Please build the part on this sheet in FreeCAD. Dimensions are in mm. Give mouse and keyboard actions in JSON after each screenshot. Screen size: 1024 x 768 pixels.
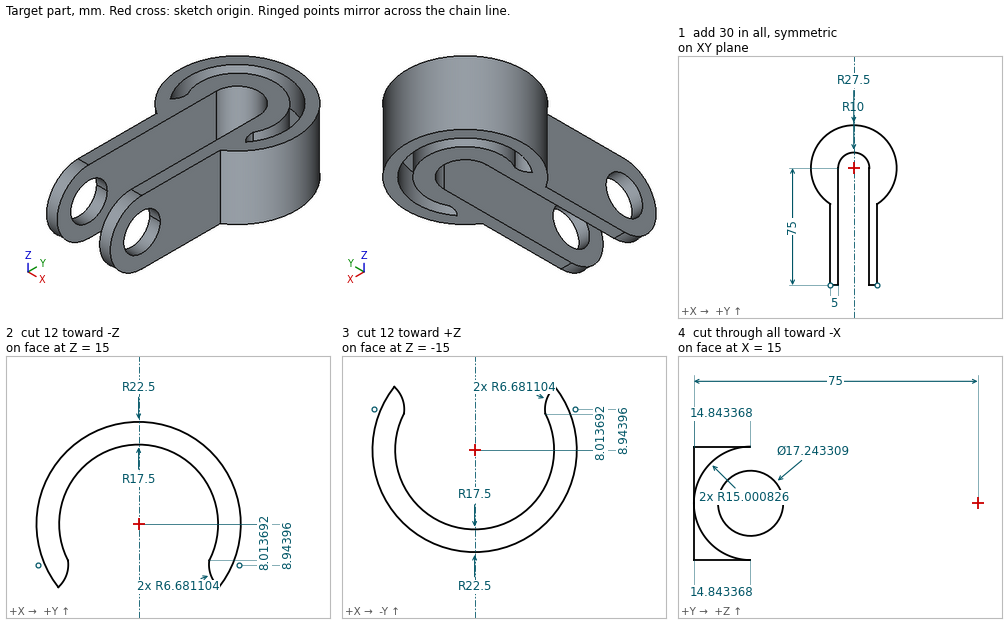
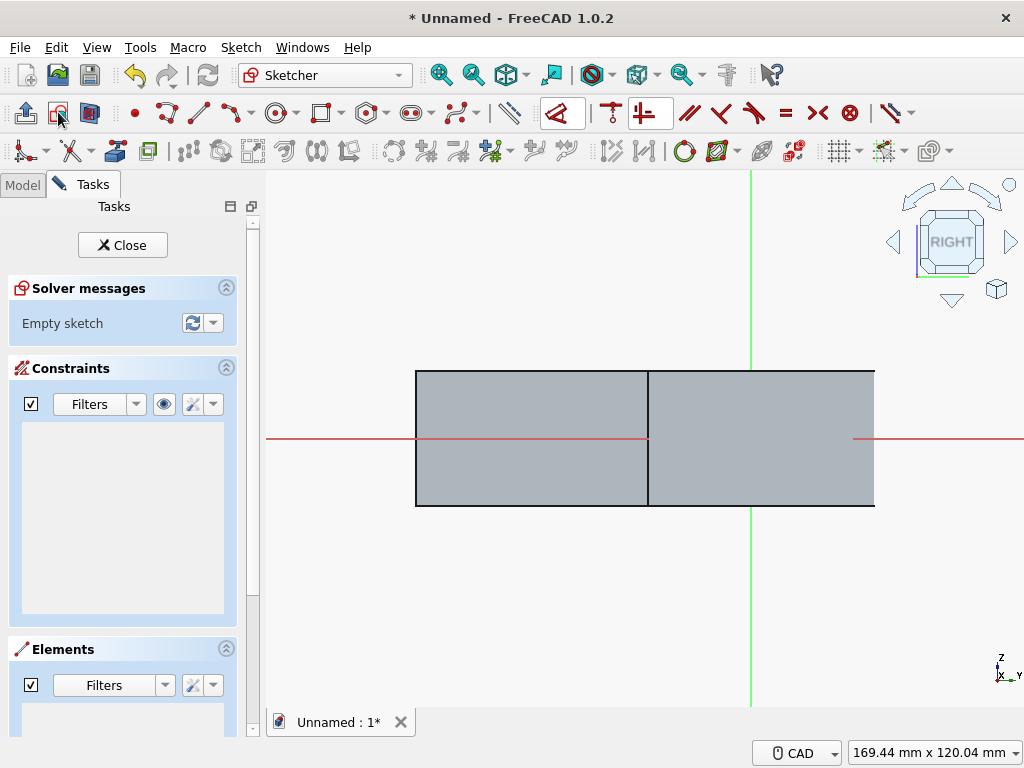
{"action": "left_click", "coordinate": [90, 114]}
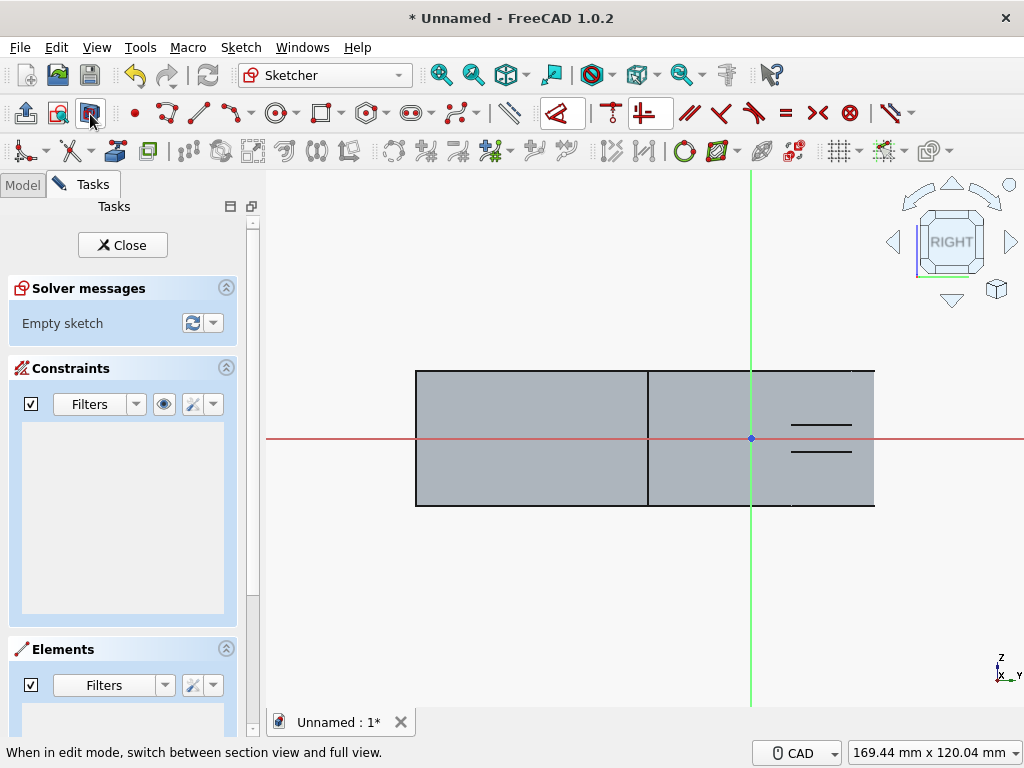
{"action": "scroll", "coordinate": [406, 439], "scroll_direction": "up", "scroll_amount": 5}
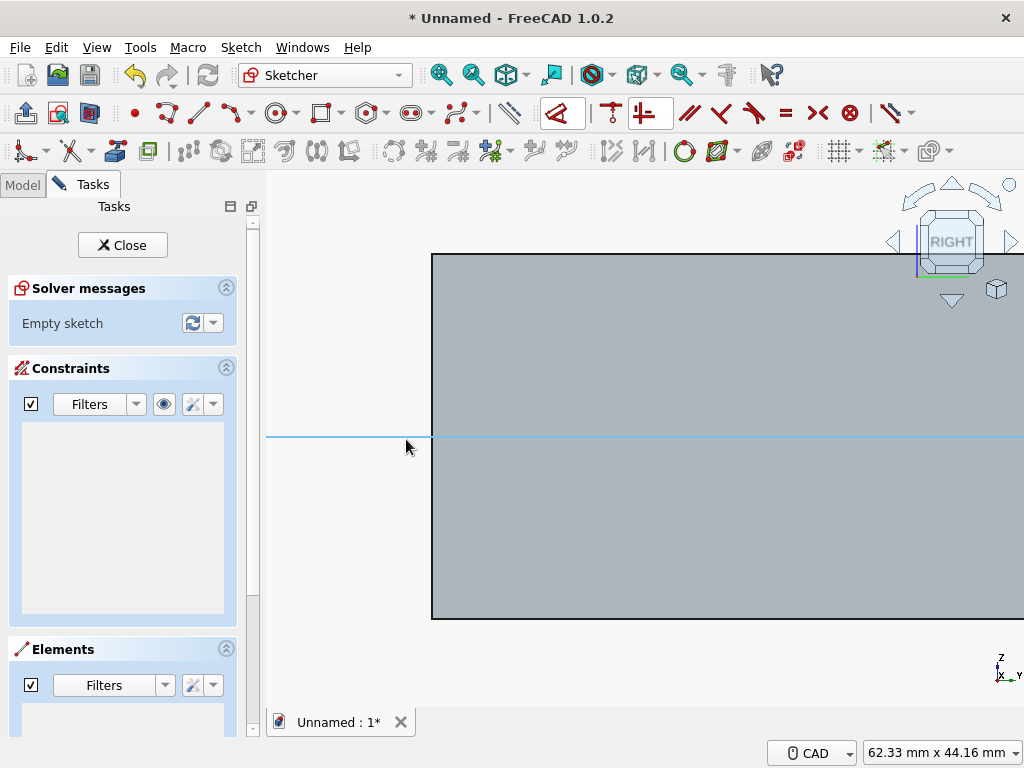
{"action": "left_click", "coordinate": [168, 114]}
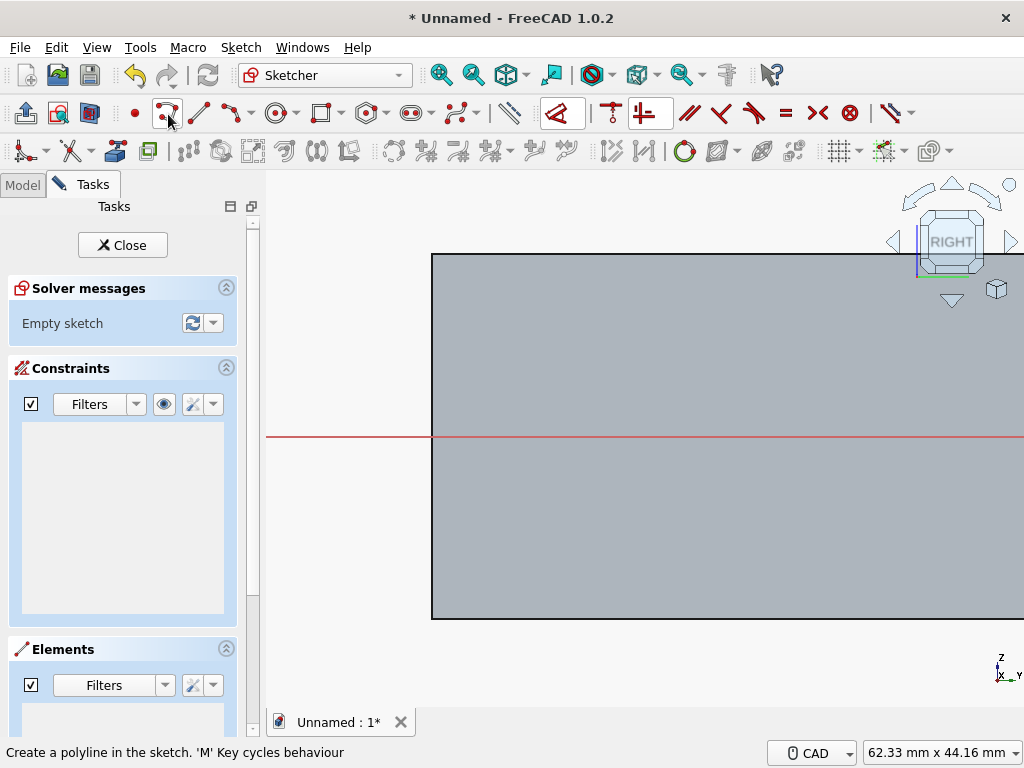
{"action": "left_click", "coordinate": [613, 254]}
{"action": "left_click", "coordinate": [432, 254]}
{"action": "left_click", "coordinate": [432, 437]}
{"action": "right_click", "coordinate": [432, 437]}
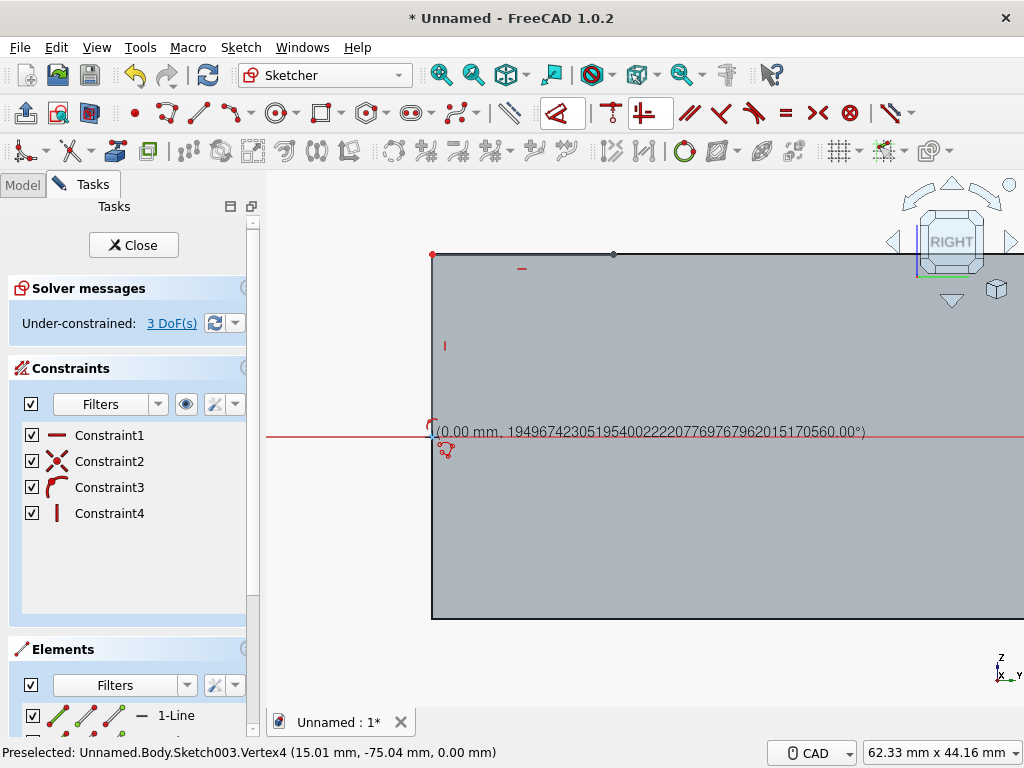
{"action": "left_click", "coordinate": [232, 114]}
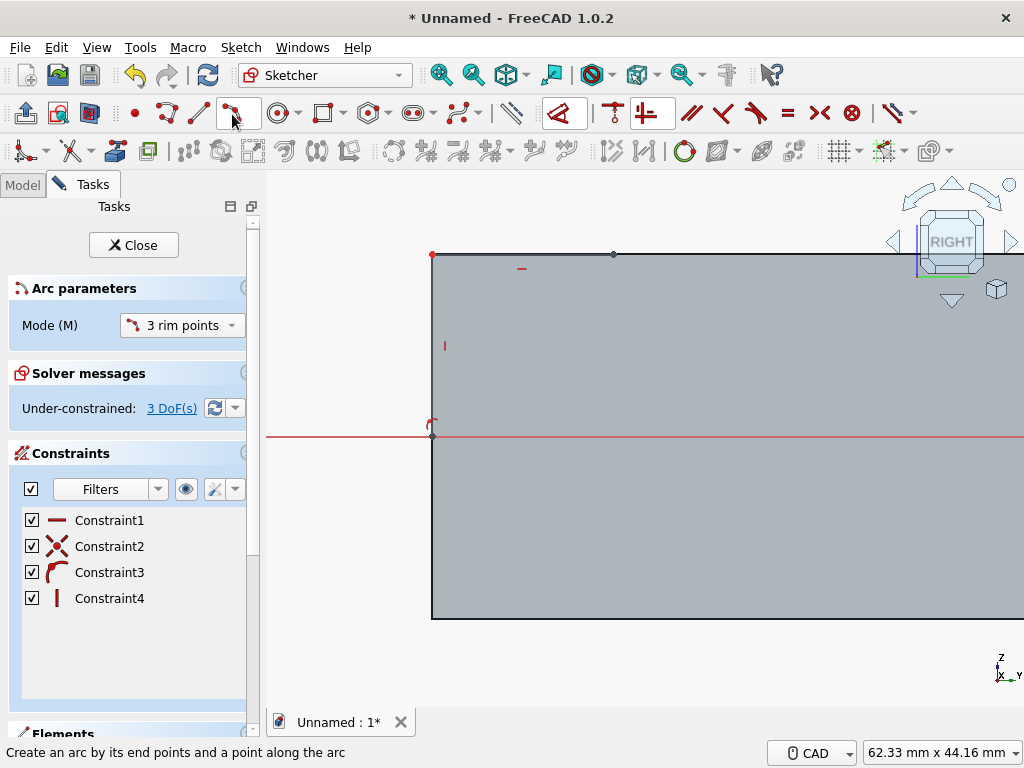
{"action": "left_click", "coordinate": [432, 437]}
{"action": "left_click", "coordinate": [613, 255]}
{"action": "left_click", "coordinate": [485, 308]}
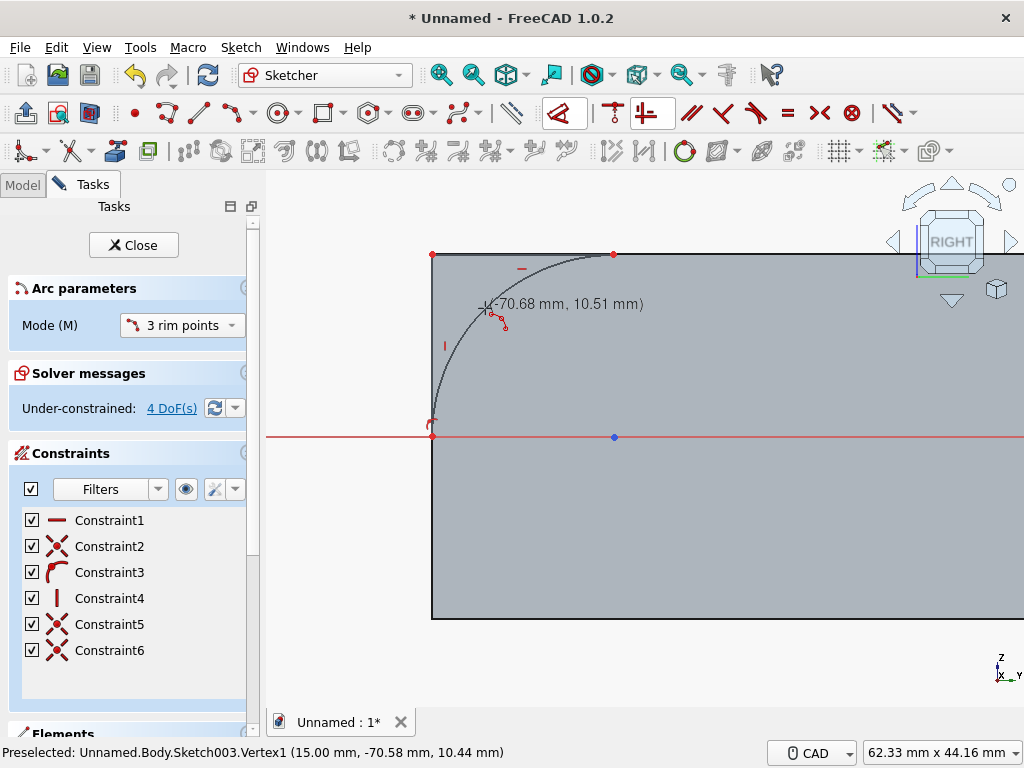
{"action": "left_click", "coordinate": [168, 114]}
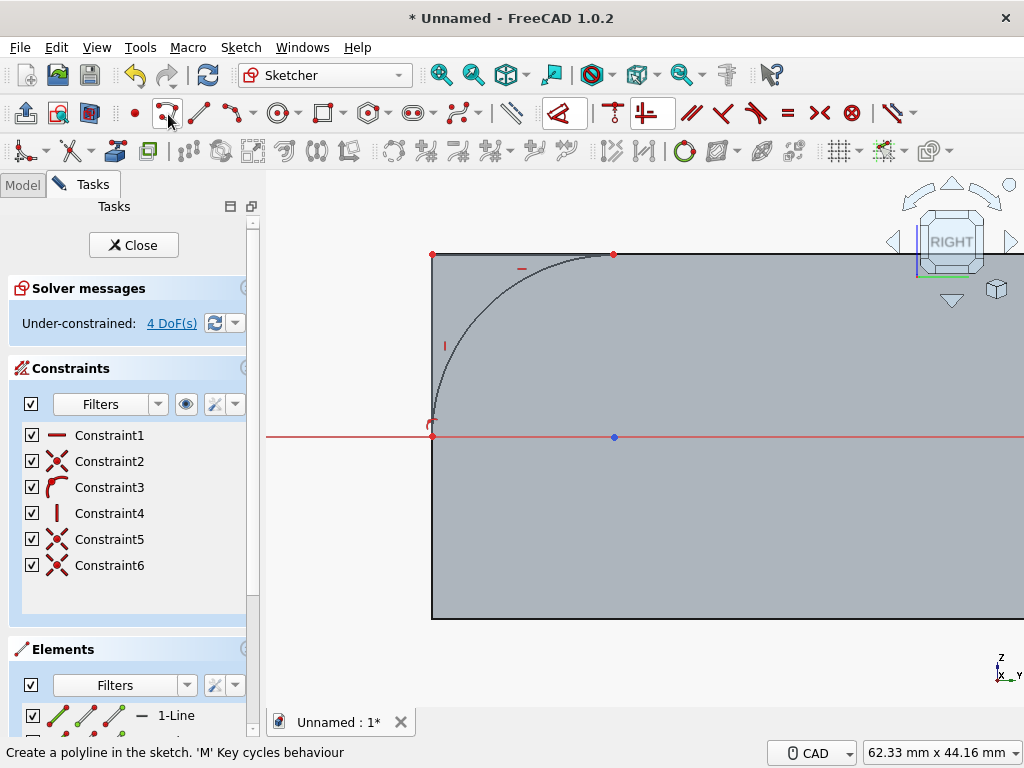
{"action": "left_click", "coordinate": [432, 437]}
{"action": "left_click", "coordinate": [432, 619]}
{"action": "left_click", "coordinate": [613, 619]}
{"action": "right_click", "coordinate": [613, 619]}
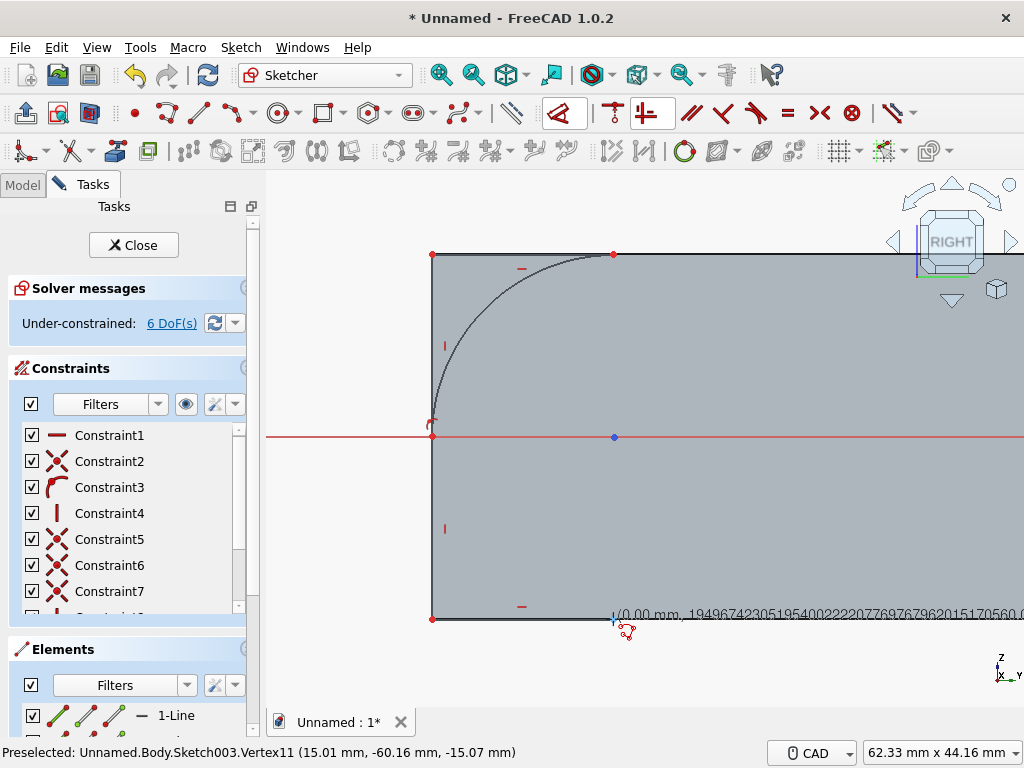
{"action": "key", "text": "g 3 a"}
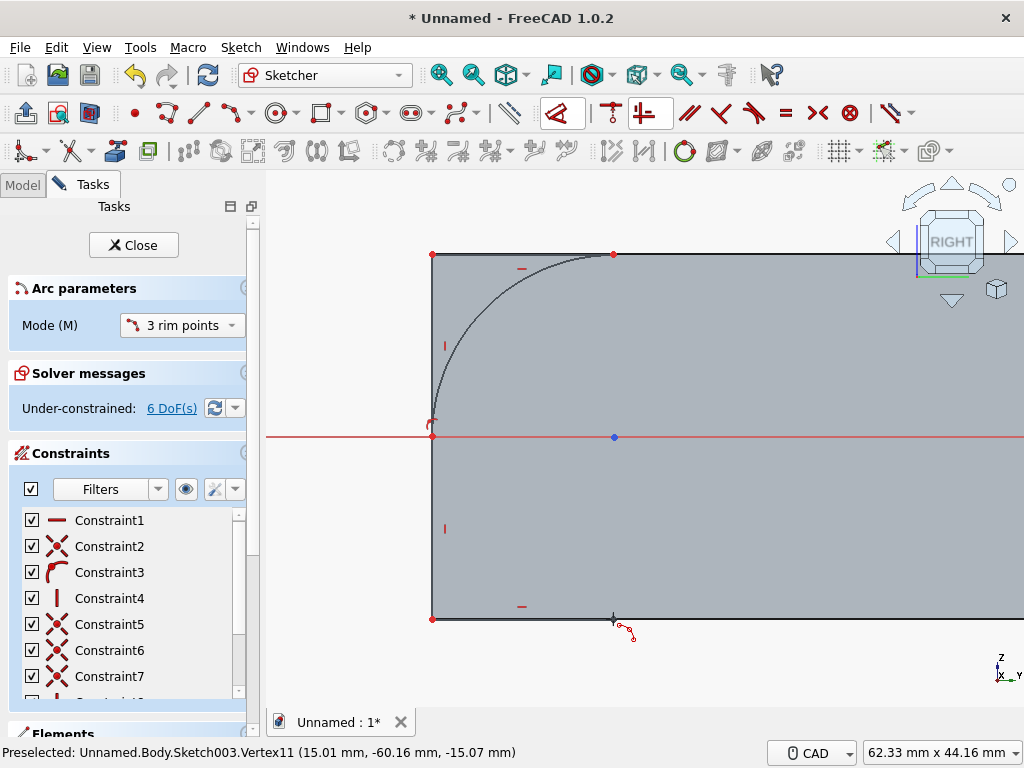
{"action": "left_click", "coordinate": [613, 620]}
{"action": "left_click", "coordinate": [432, 437]}
{"action": "left_click", "coordinate": [485, 565]}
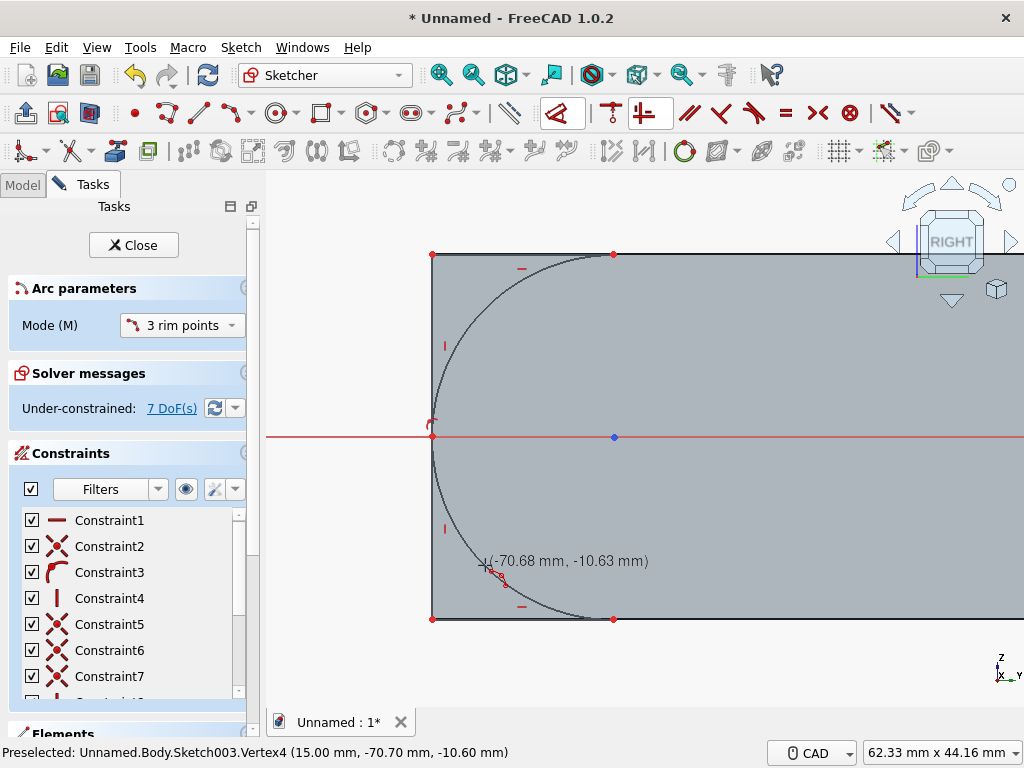
{"action": "left_click", "coordinate": [276, 114]}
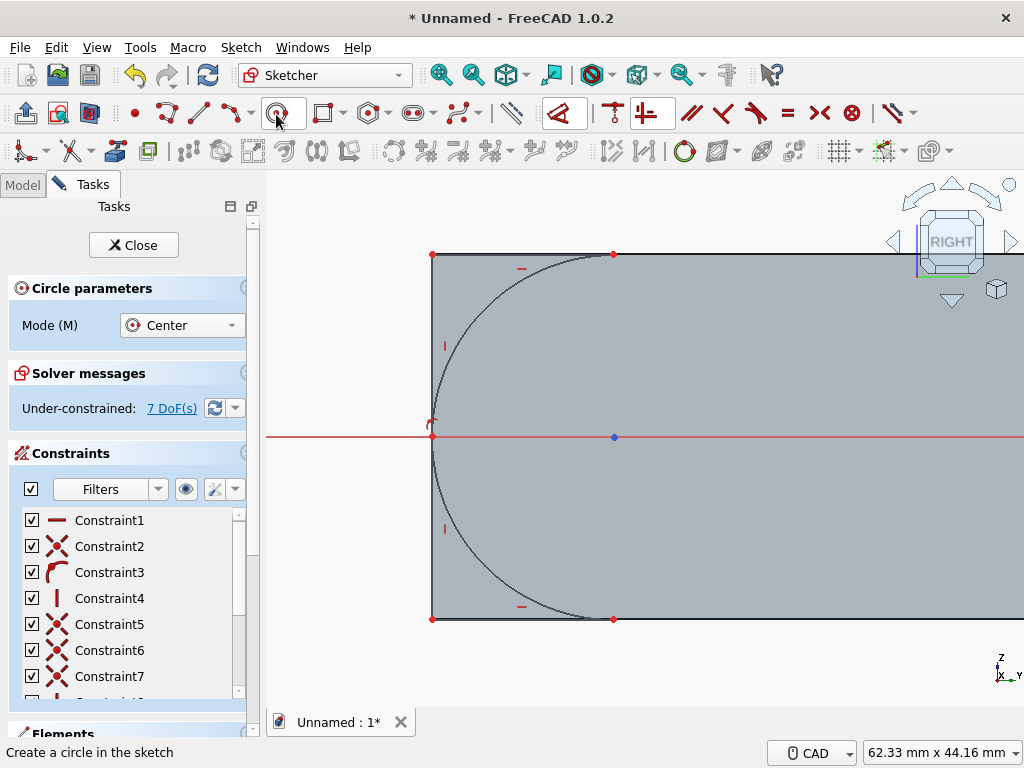
{"action": "left_click", "coordinate": [615, 437]}
{"action": "left_click", "coordinate": [689, 363]}
{"action": "key", "text": "Escape"}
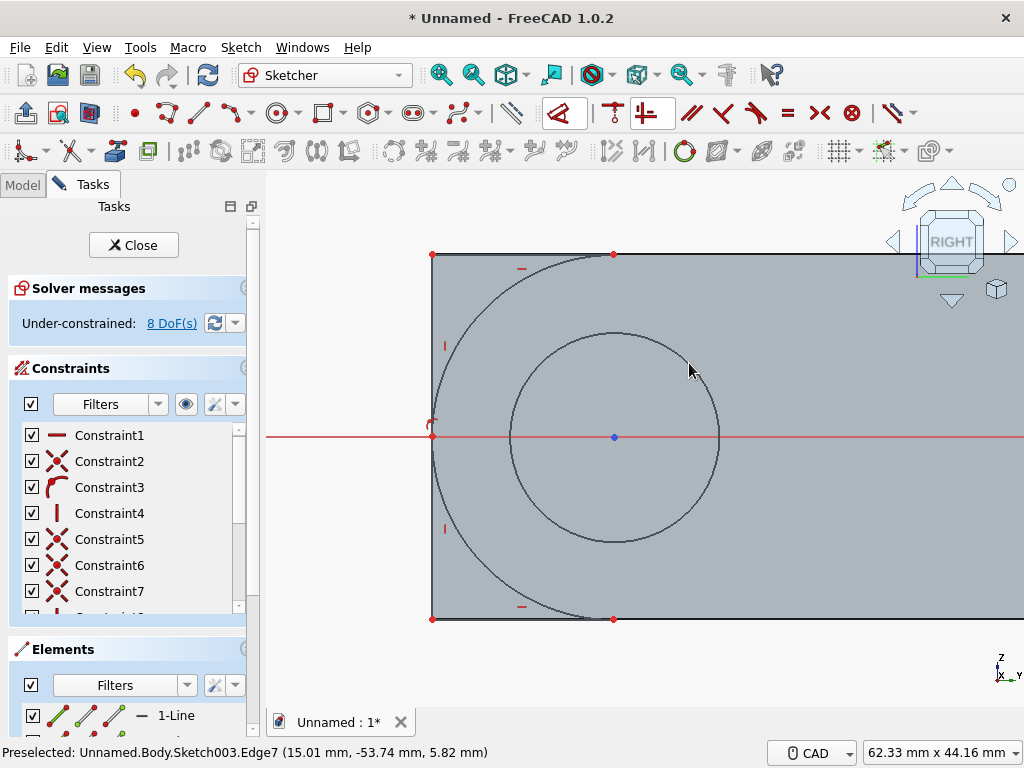
{"action": "left_click", "coordinate": [432, 310]}